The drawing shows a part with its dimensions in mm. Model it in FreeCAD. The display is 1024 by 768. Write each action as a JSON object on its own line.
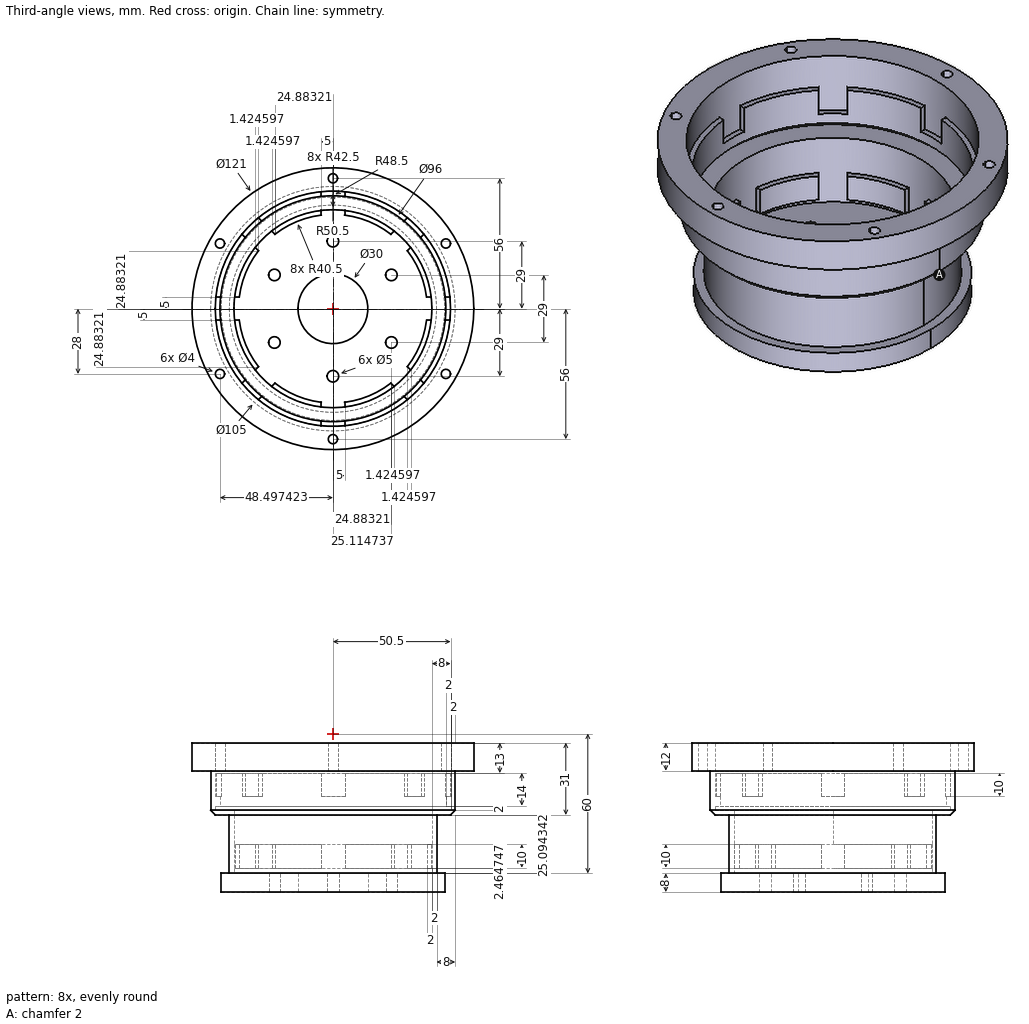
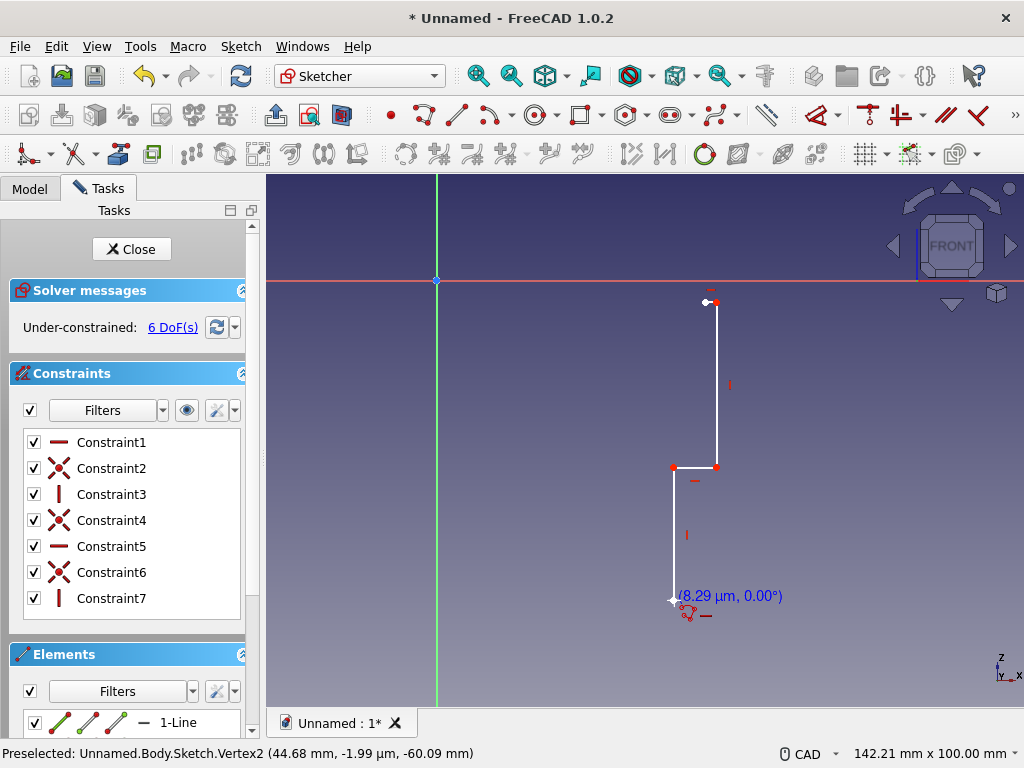
{"action": "scroll", "coordinate": [663, 600], "scroll_direction": "up", "scroll_amount": 2}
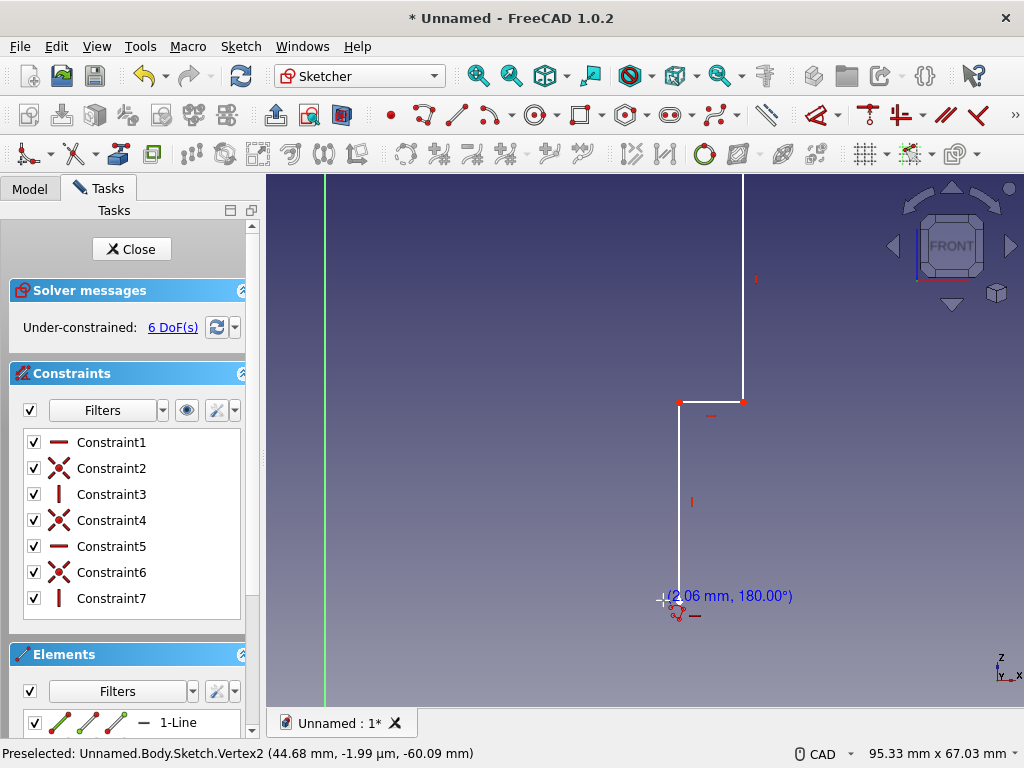
{"action": "left_click", "coordinate": [663, 600]}
{"action": "left_click", "coordinate": [663, 581]}
{"action": "left_click", "coordinate": [647, 581]}
{"action": "left_click", "coordinate": [647, 501]}
{"action": "left_click", "coordinate": [663, 501]}
{"action": "left_click", "coordinate": [663, 385]}
{"action": "left_click", "coordinate": [727, 385]}
{"action": "left_click", "coordinate": [727, 369]}
{"action": "left_click", "coordinate": [711, 369]}
{"action": "left_click", "coordinate": [711, 258]}
{"action": "left_click", "coordinate": [727, 258]}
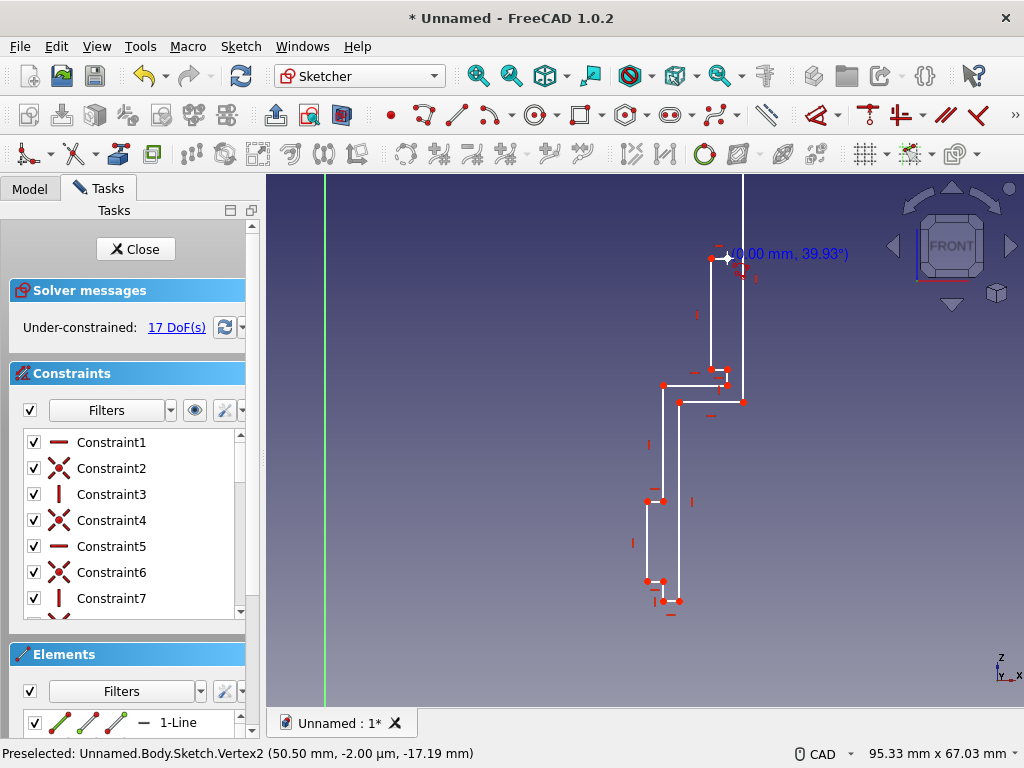
{"action": "scroll", "coordinate": [663, 601], "scroll_direction": "down", "scroll_amount": 2}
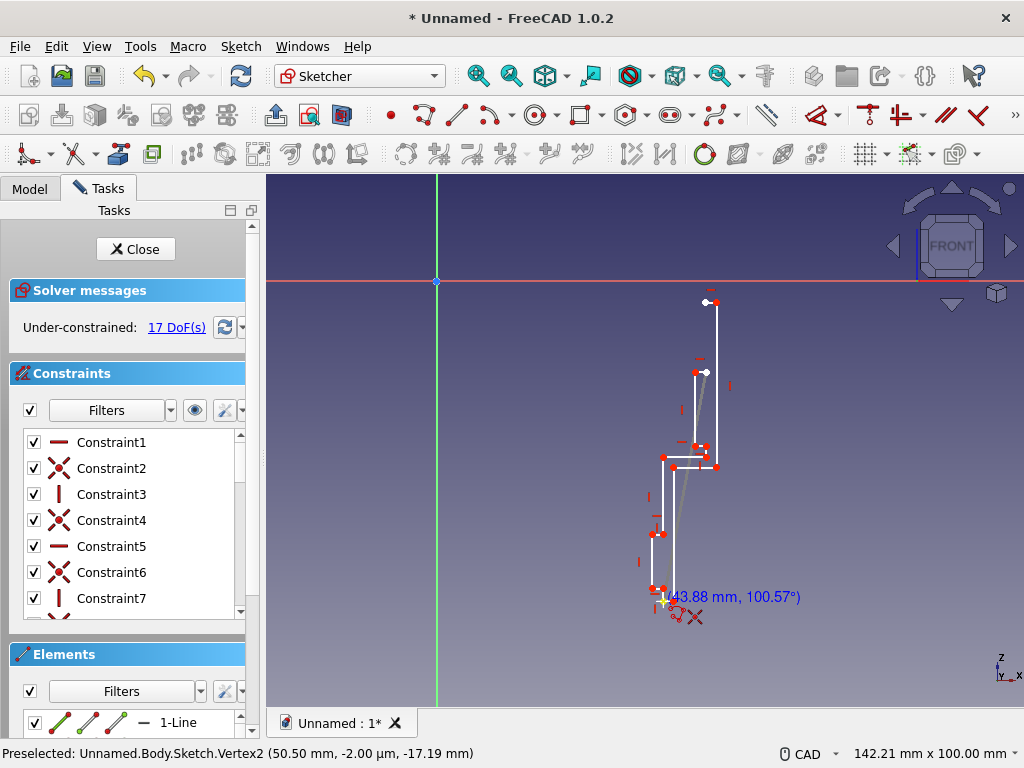
{"action": "scroll", "coordinate": [706, 302], "scroll_direction": "up", "scroll_amount": 6}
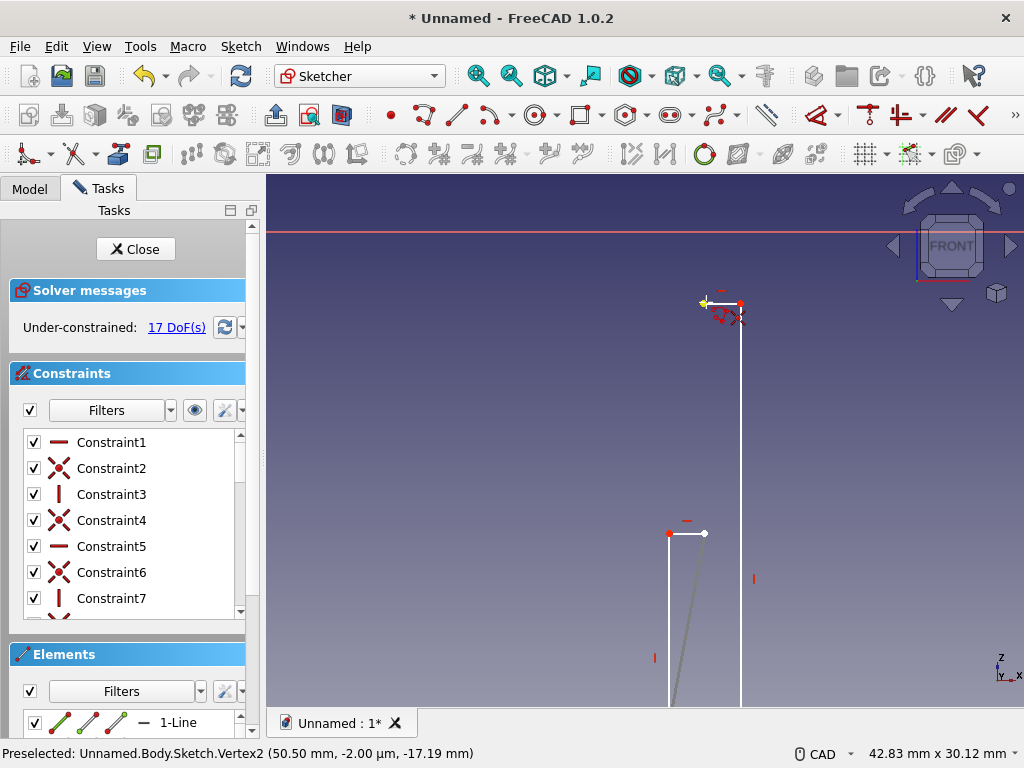
{"action": "left_click", "coordinate": [704, 304]}
{"action": "key", "text": "Escape"}
{"action": "key", "text": "Escape"}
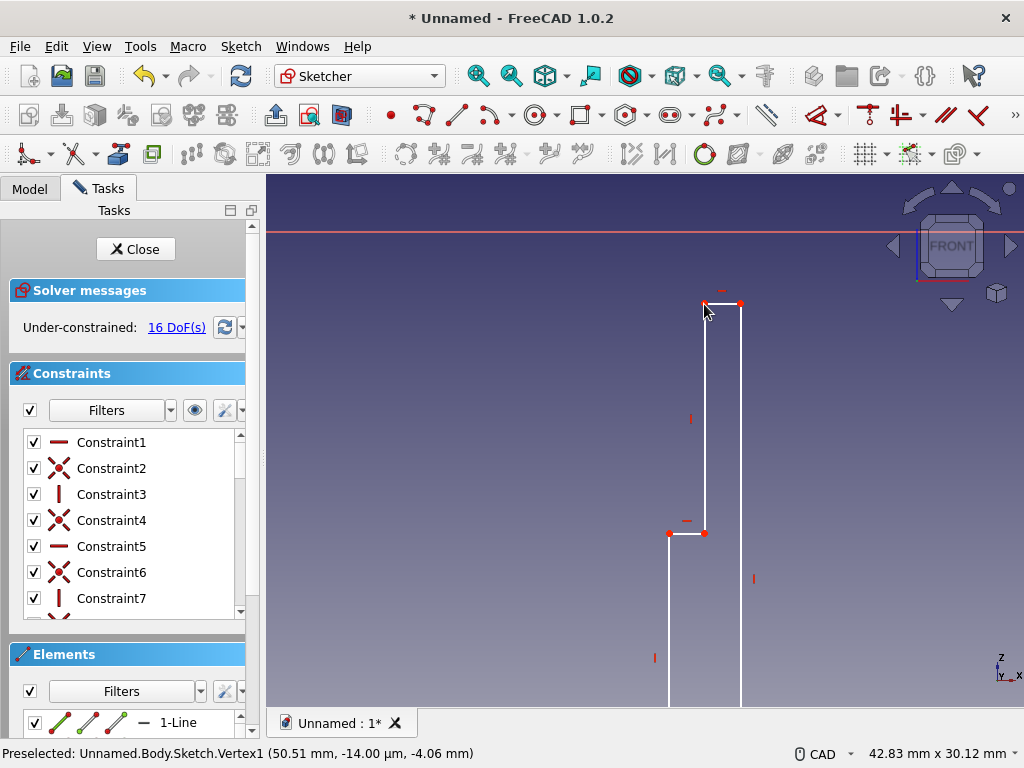
{"action": "key", "text": "d"}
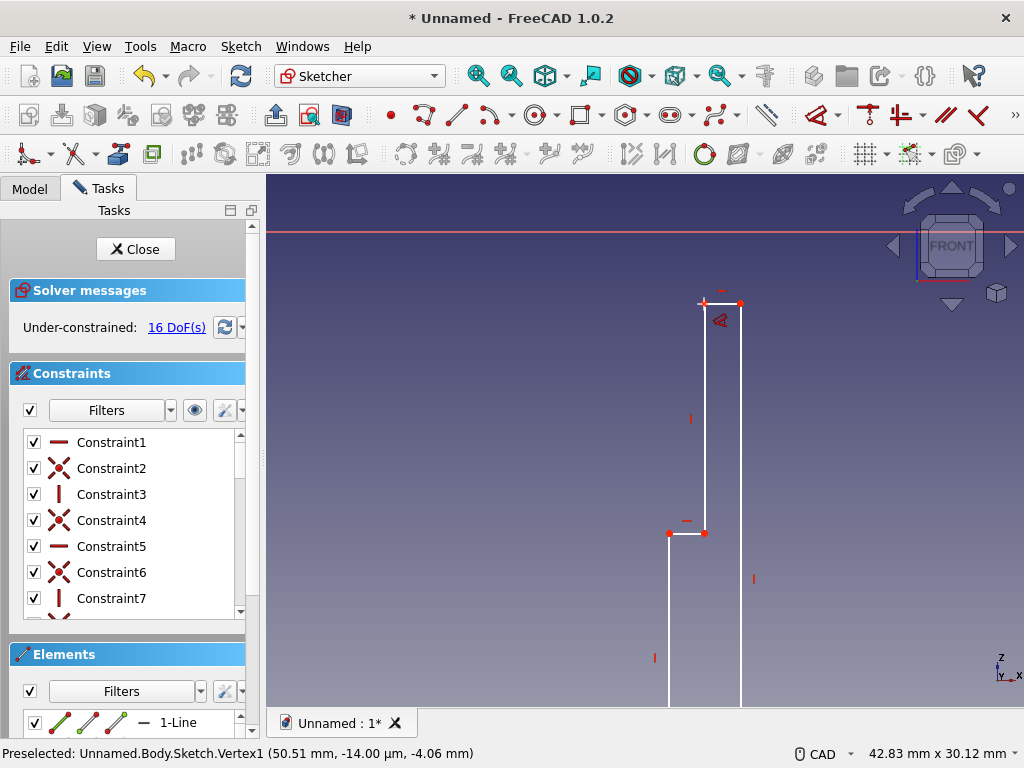
{"action": "scroll", "coordinate": [716, 304], "scroll_direction": "up", "scroll_amount": 2}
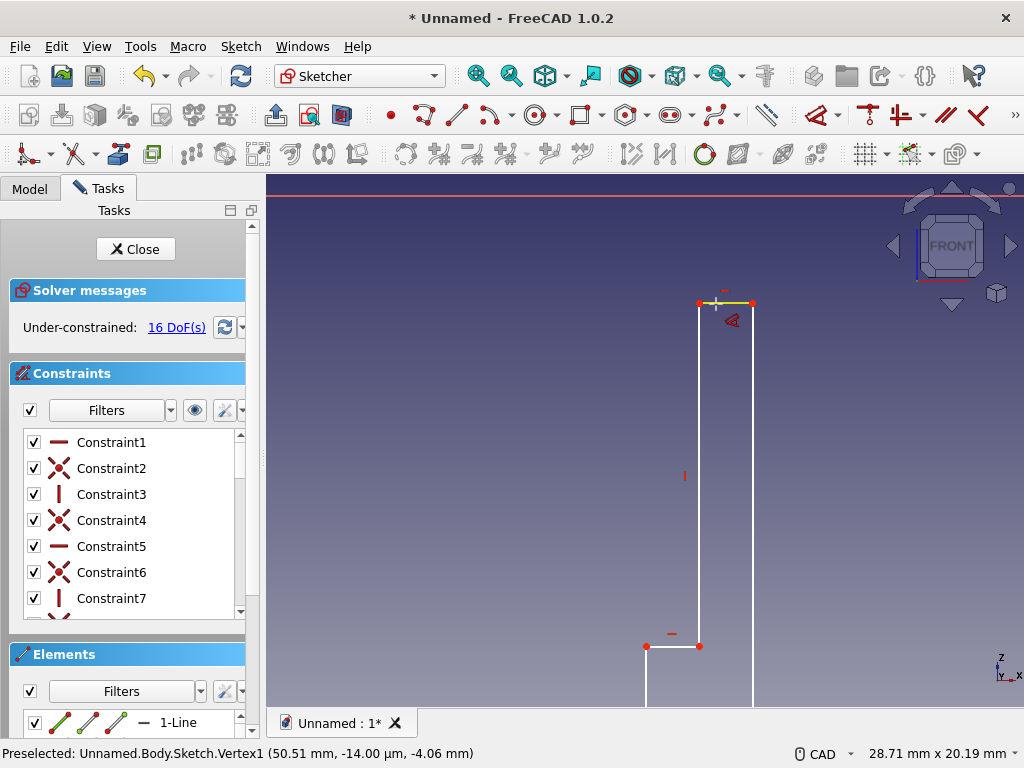
{"action": "left_click", "coordinate": [715, 303]}
{"action": "left_click", "coordinate": [726, 269]}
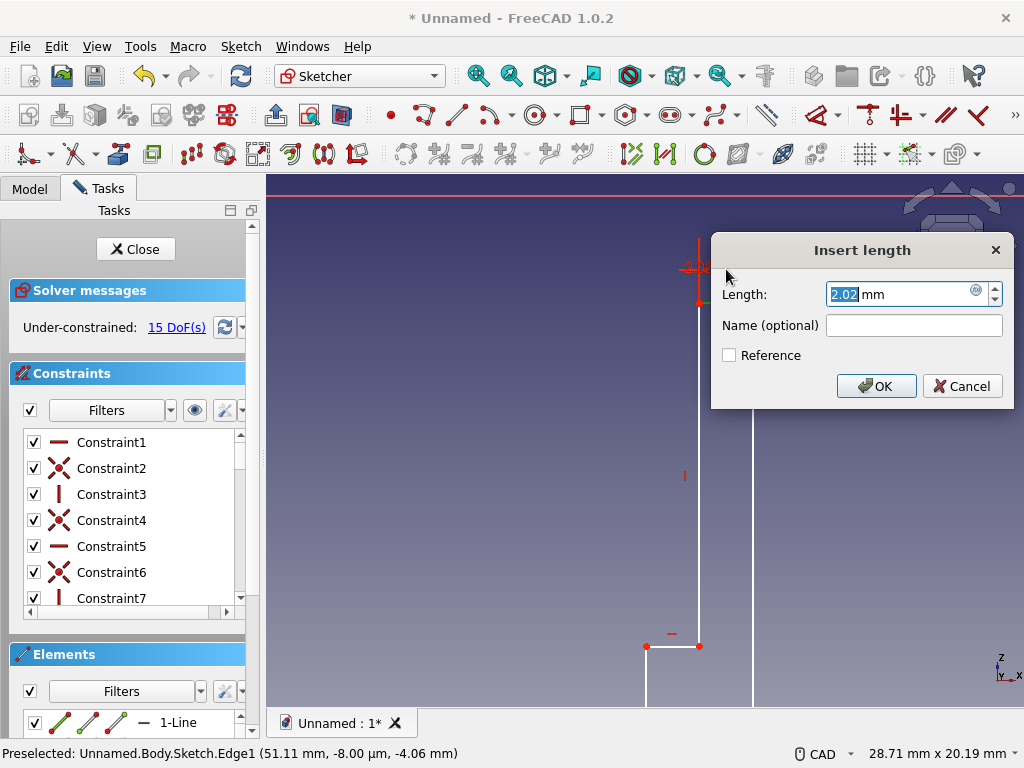
{"action": "type", "text": "2"}
{"action": "key", "text": "Return"}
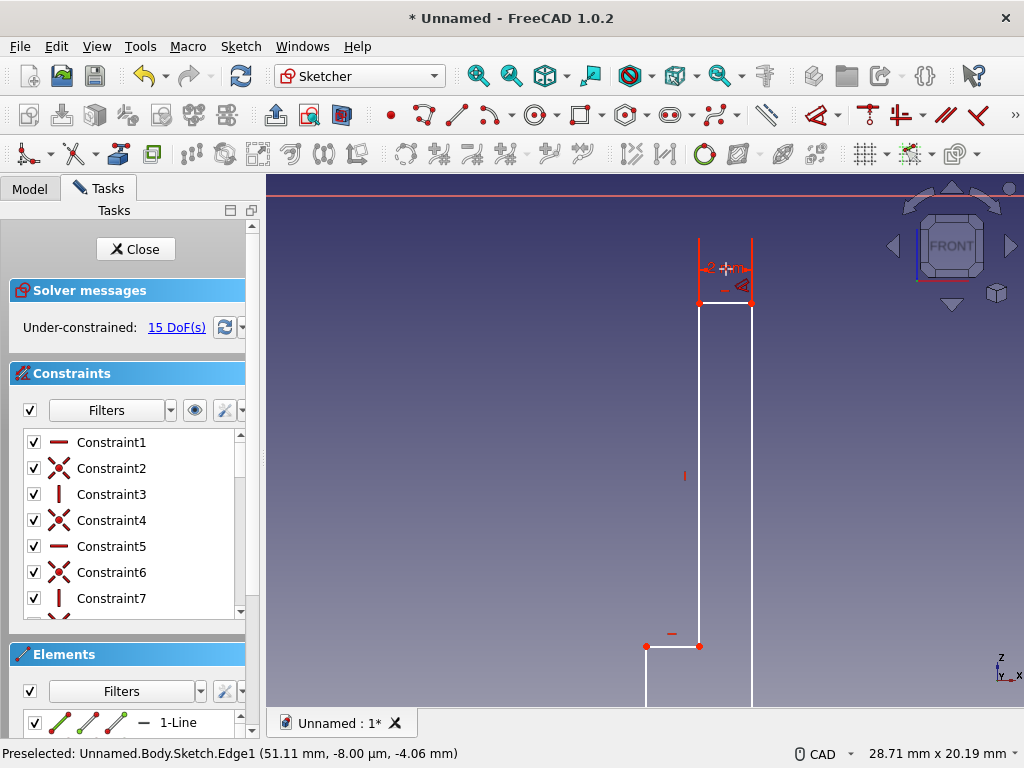
{"action": "scroll", "coordinate": [707, 302], "scroll_direction": "down", "scroll_amount": 8}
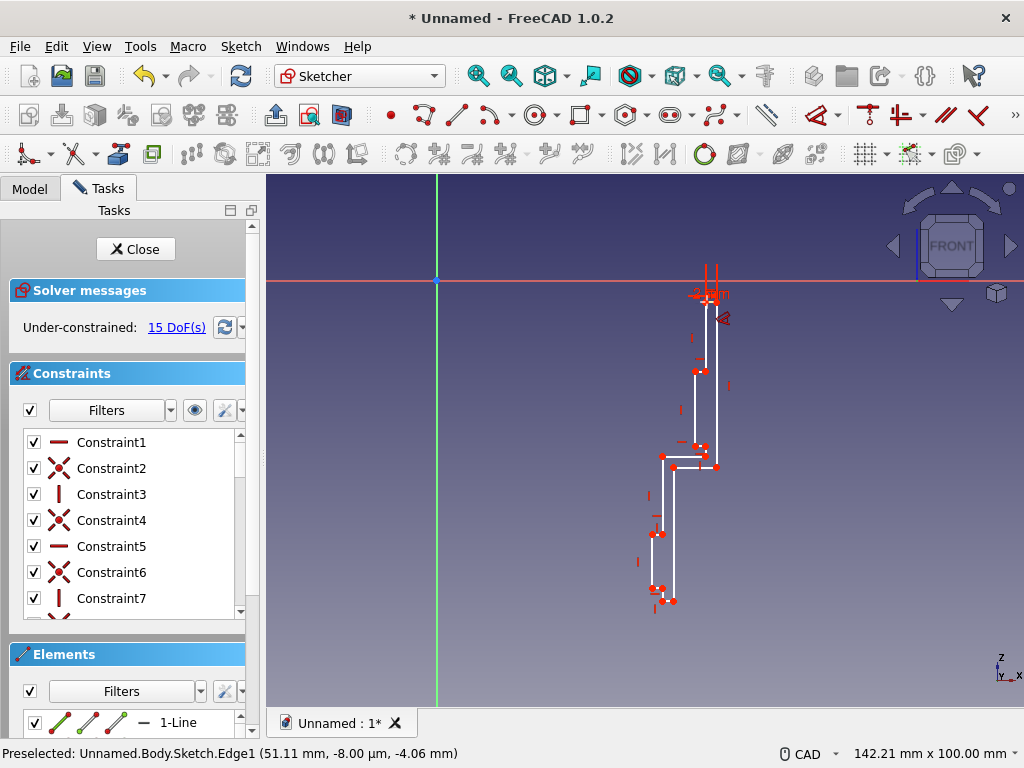
{"action": "scroll", "coordinate": [704, 468], "scroll_direction": "up", "scroll_amount": 2}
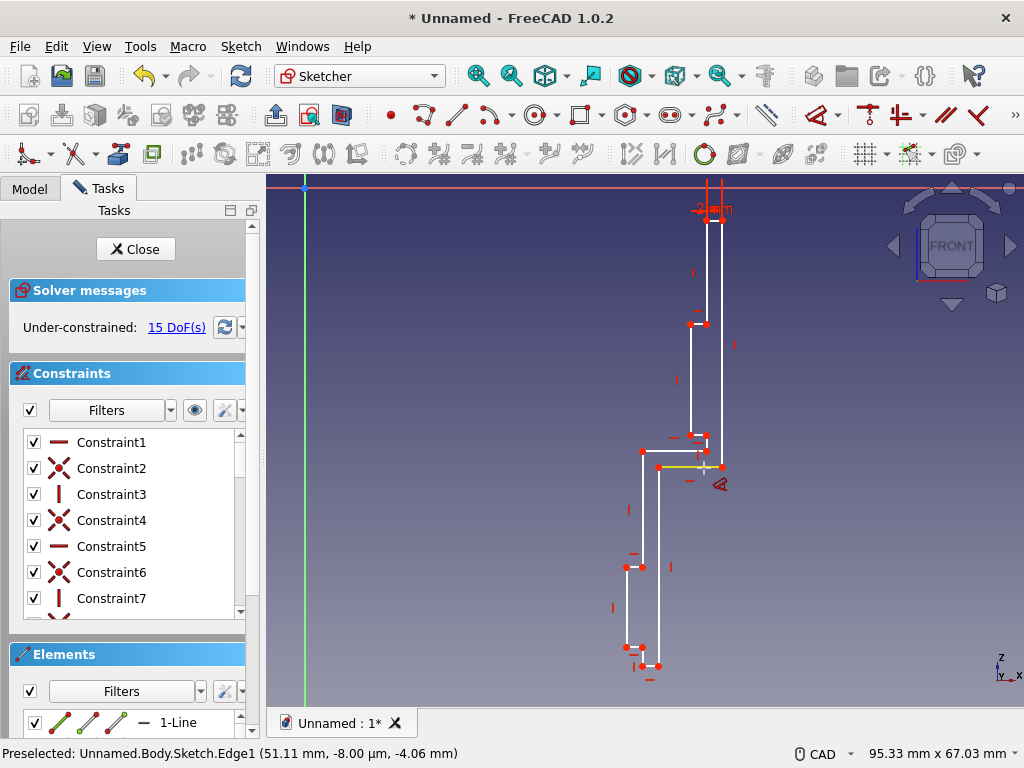
{"action": "left_click", "coordinate": [703, 467]}
{"action": "left_click", "coordinate": [691, 501]}